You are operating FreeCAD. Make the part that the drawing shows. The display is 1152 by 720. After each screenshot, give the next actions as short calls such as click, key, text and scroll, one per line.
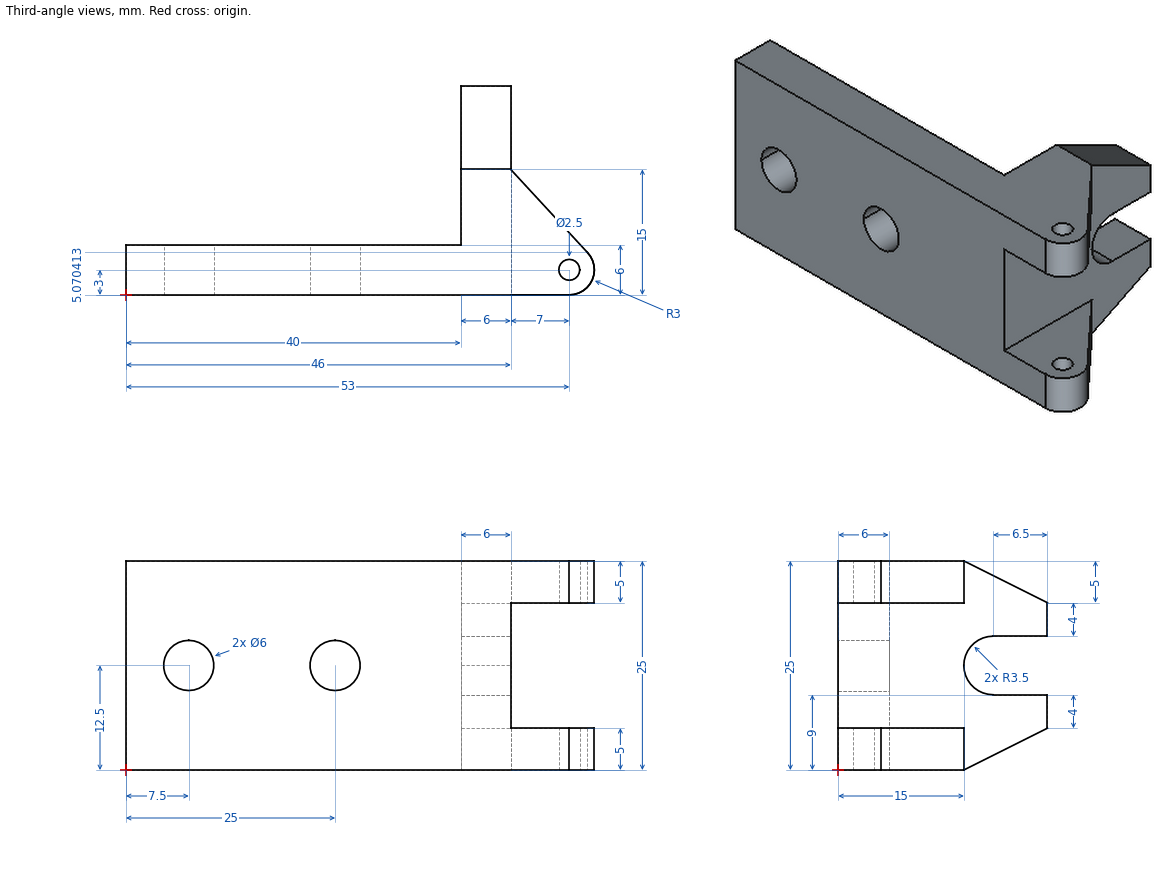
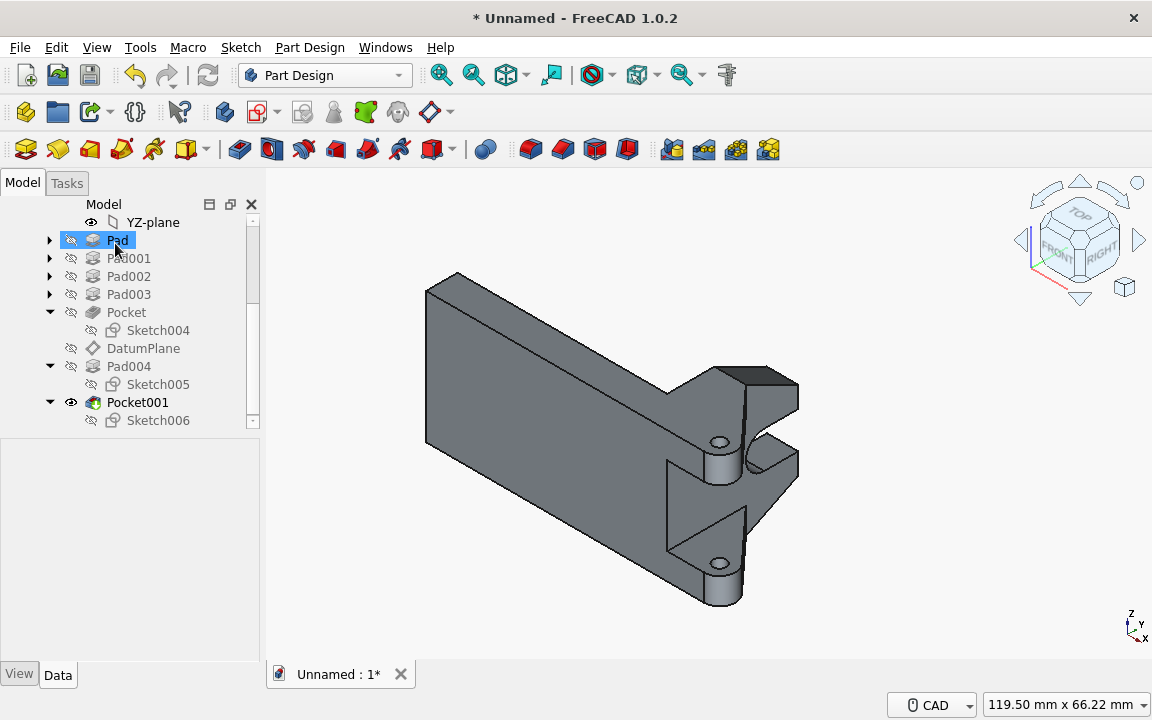
key(4)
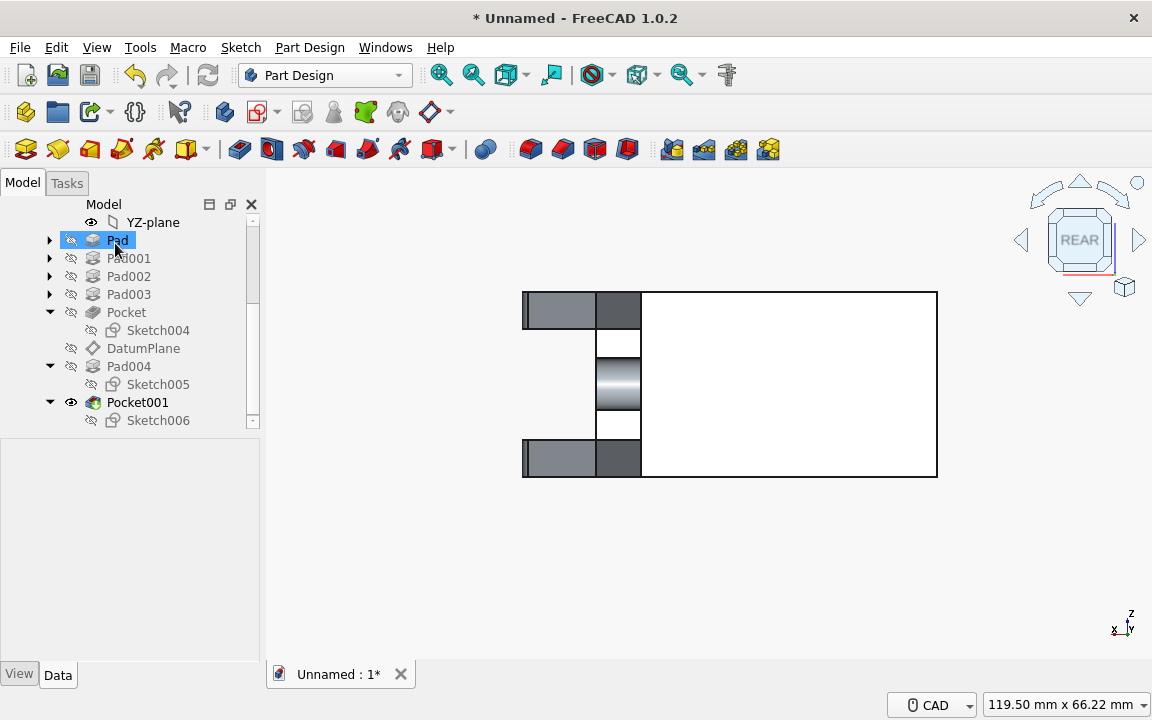
click(747, 383)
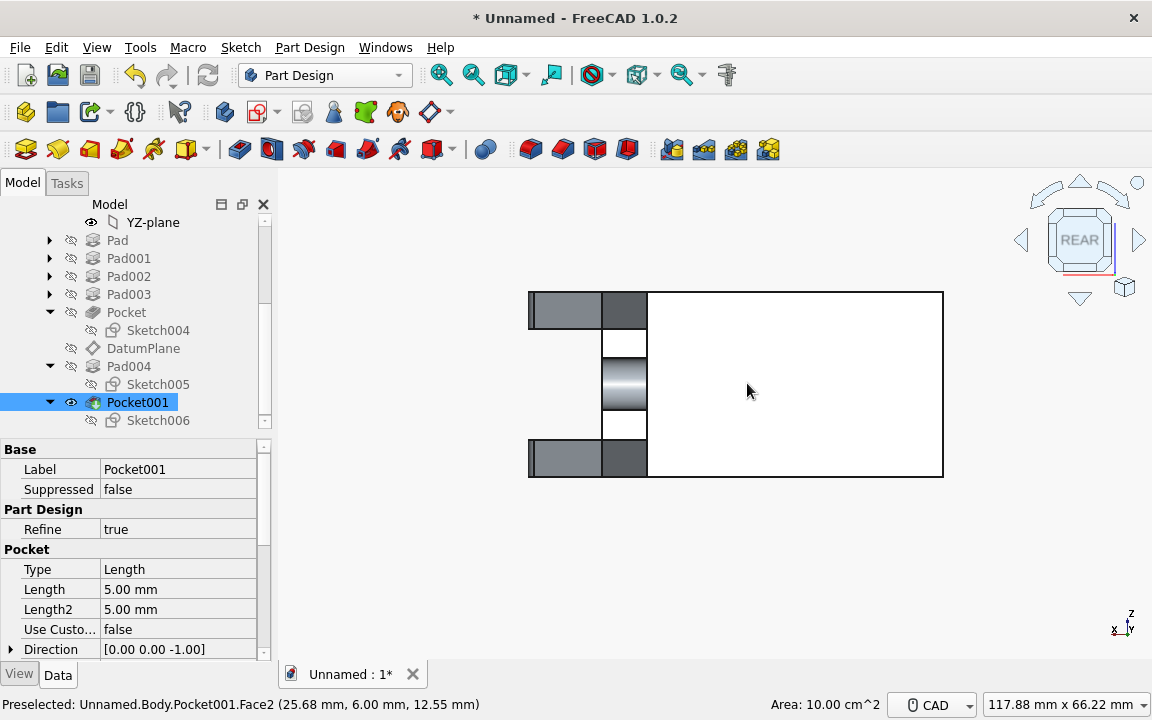
click(258, 112)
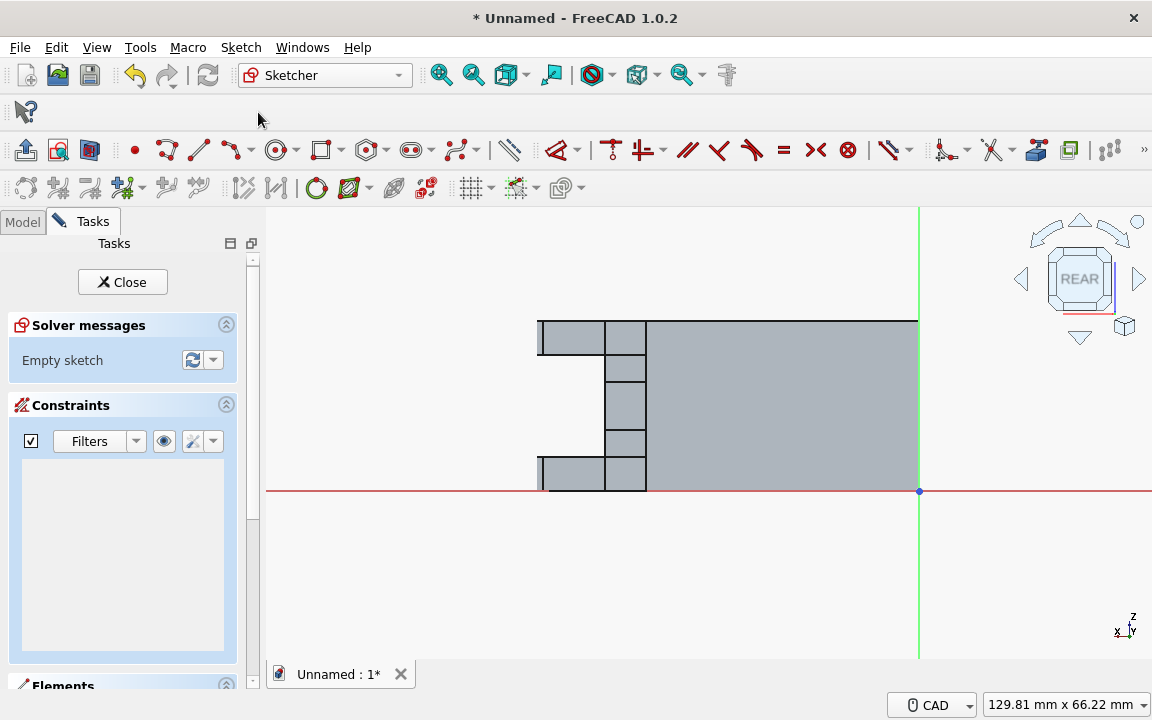
scroll(930, 442, up, 5)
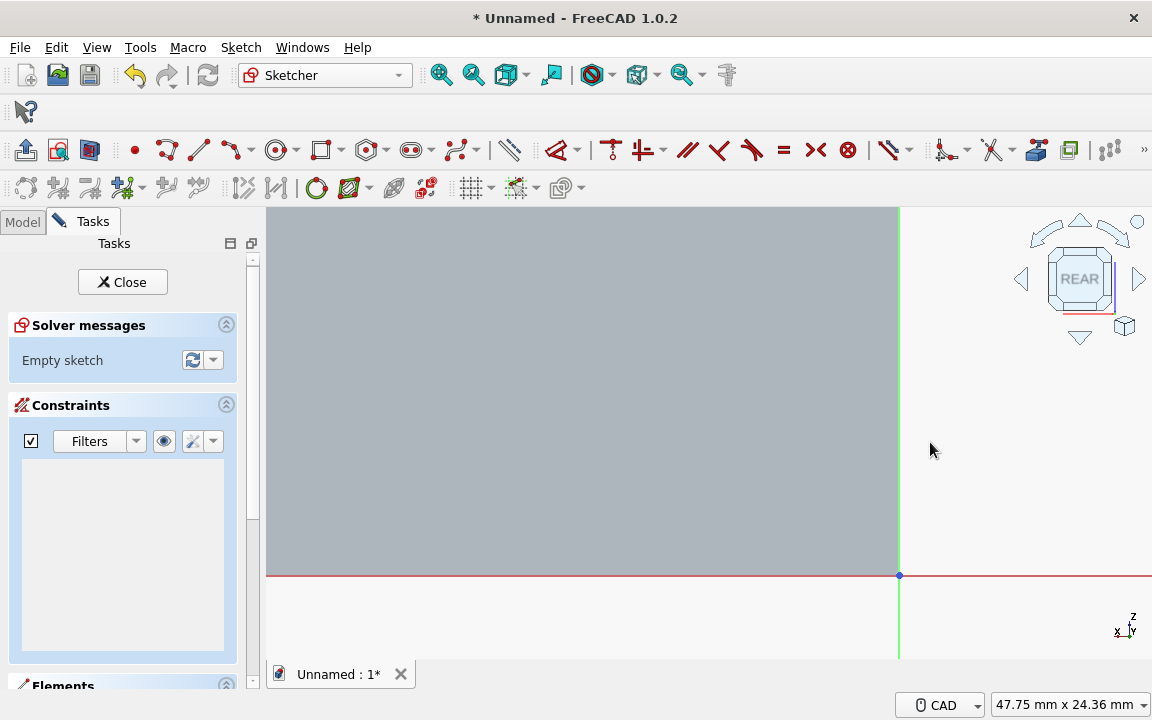
key(g)
key(c)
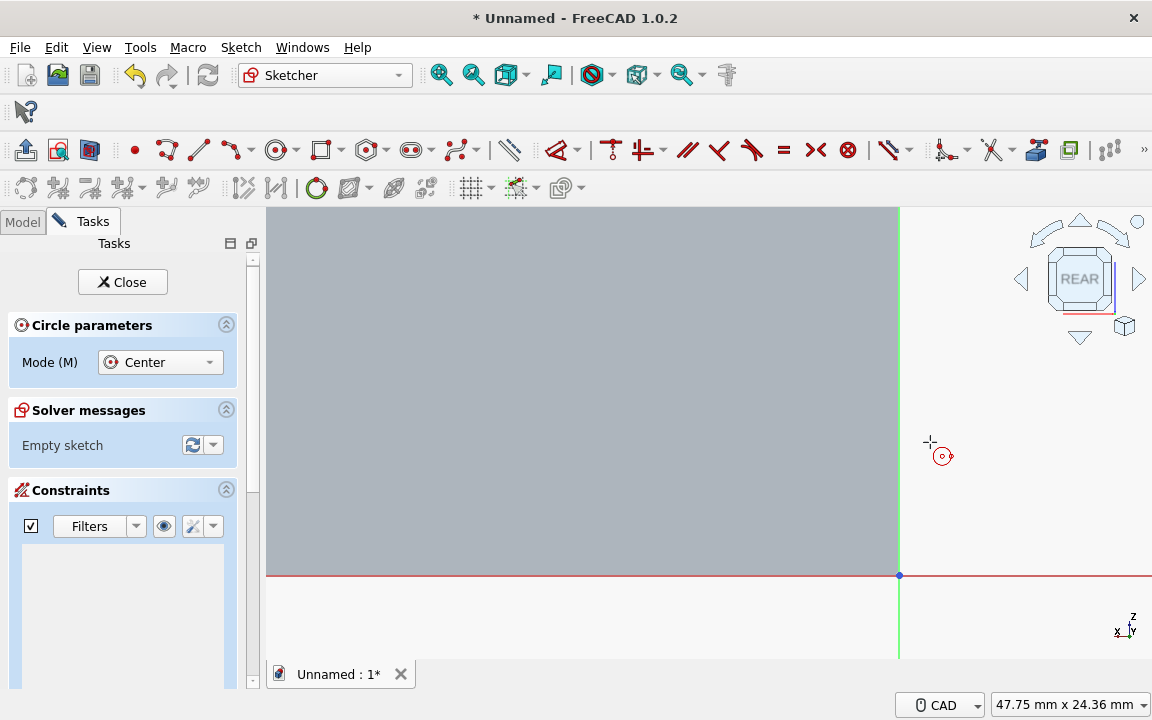
click(760, 344)
click(800, 304)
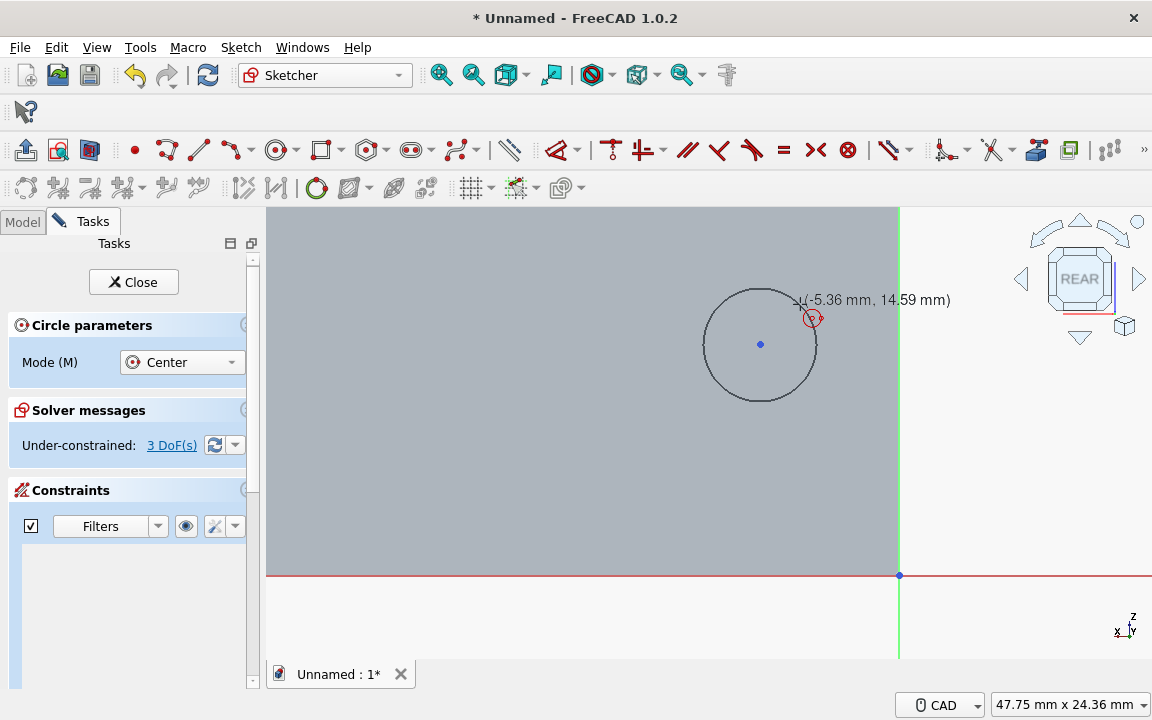
click(436, 344)
click(475, 304)
key(Escape)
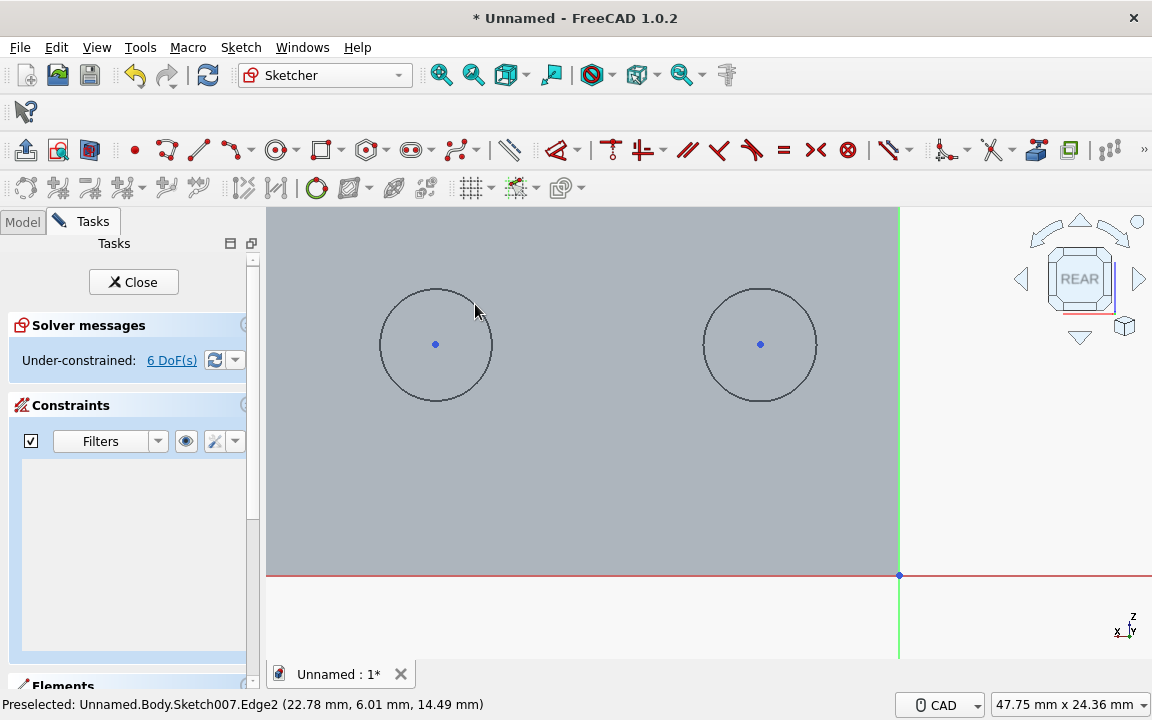
click(800, 305)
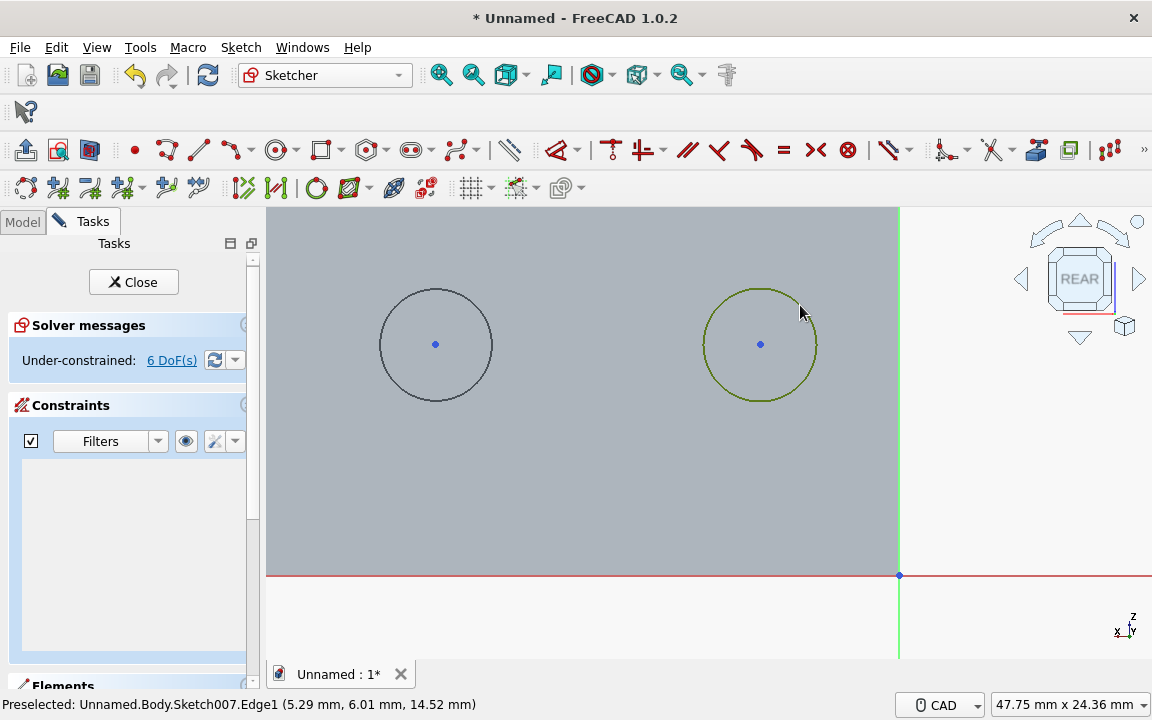
click(475, 305)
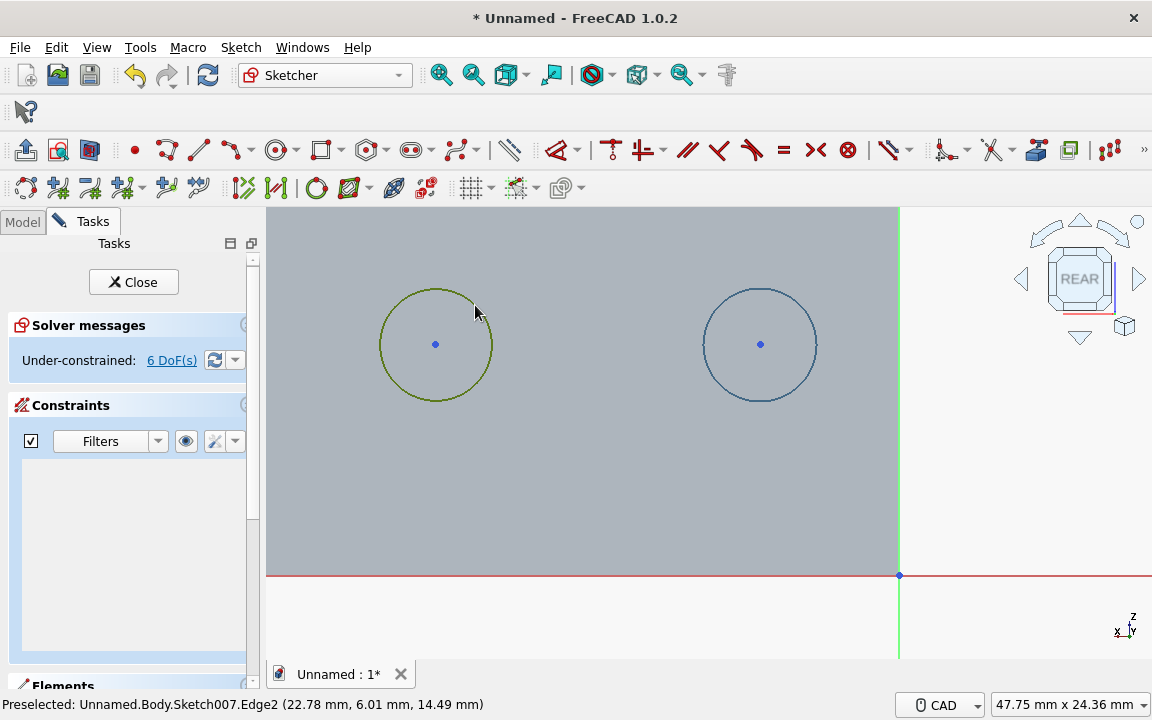
click(784, 150)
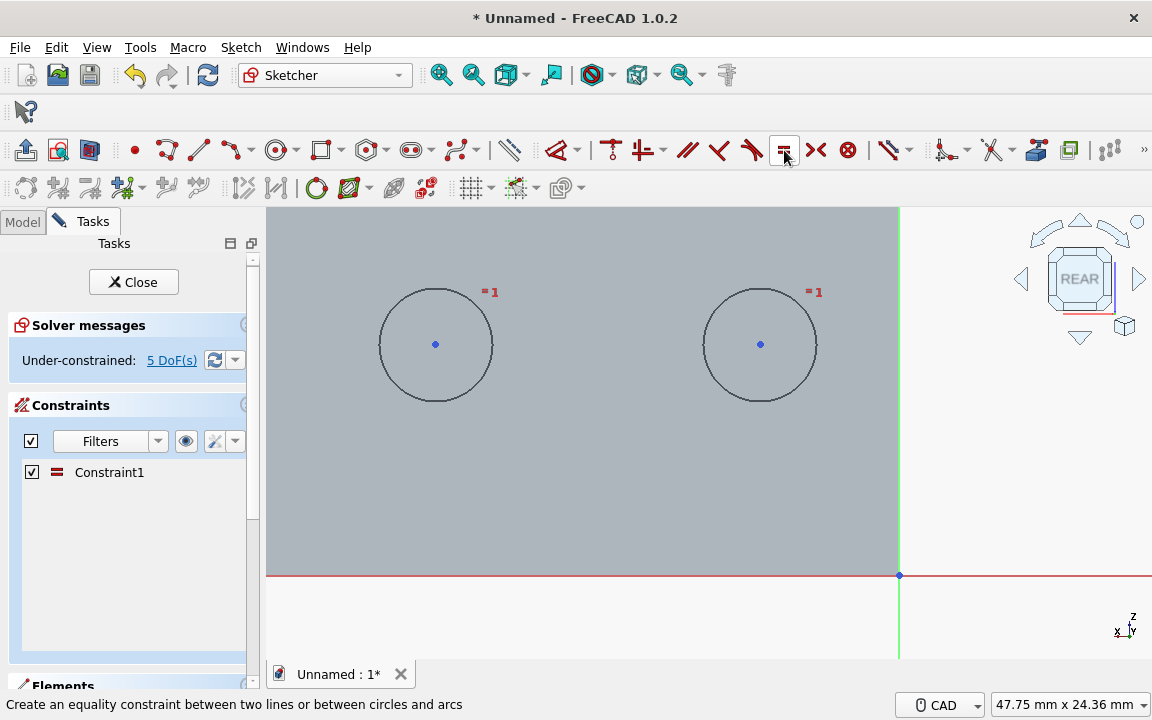
click(760, 345)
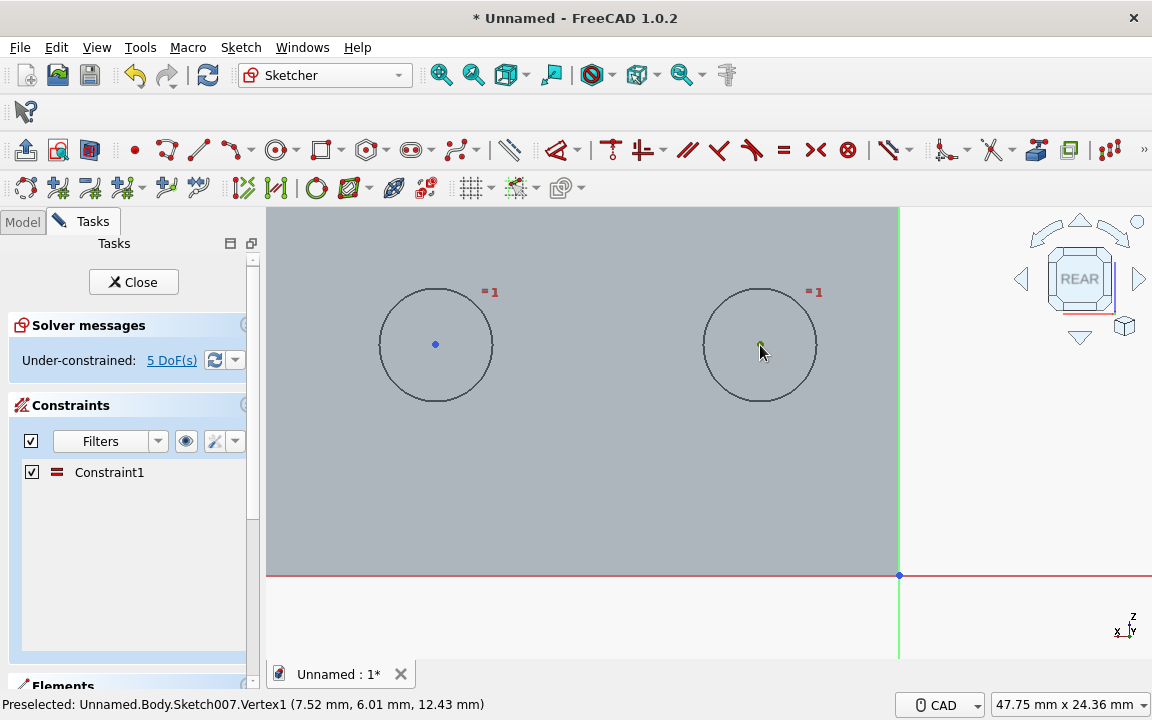
click(436, 345)